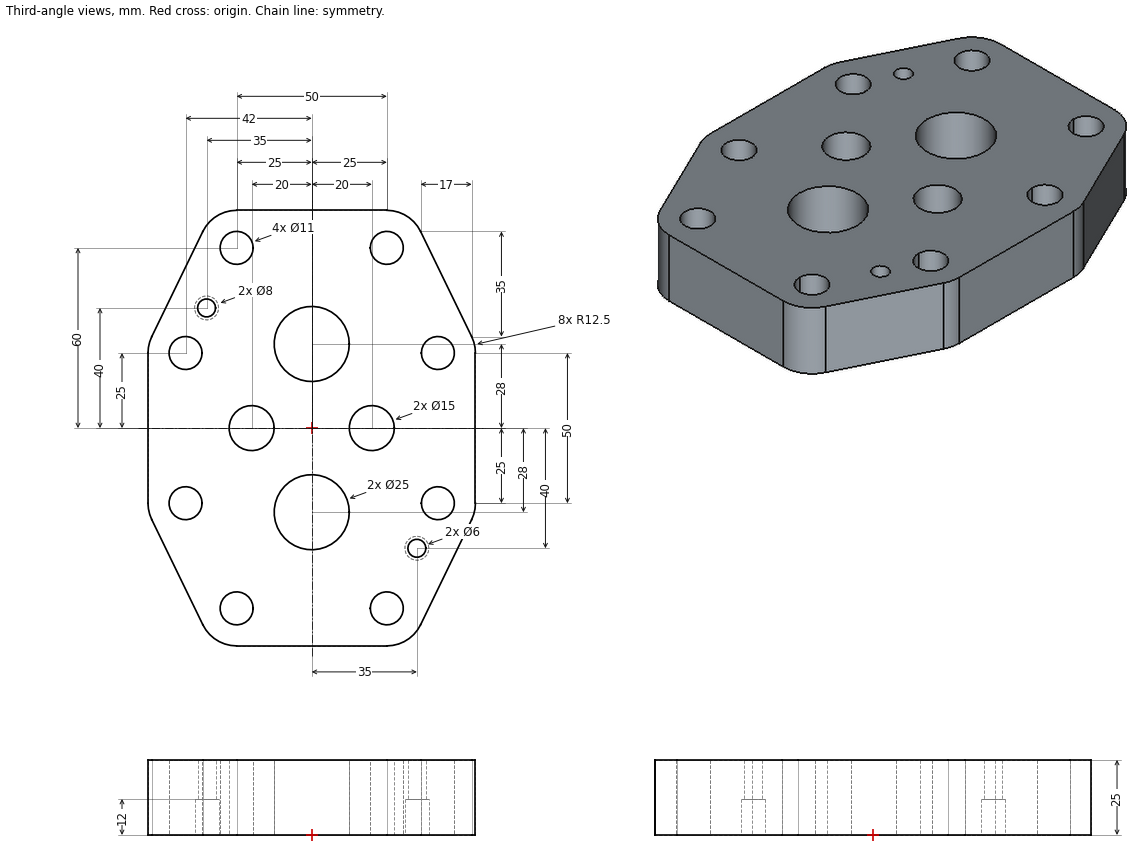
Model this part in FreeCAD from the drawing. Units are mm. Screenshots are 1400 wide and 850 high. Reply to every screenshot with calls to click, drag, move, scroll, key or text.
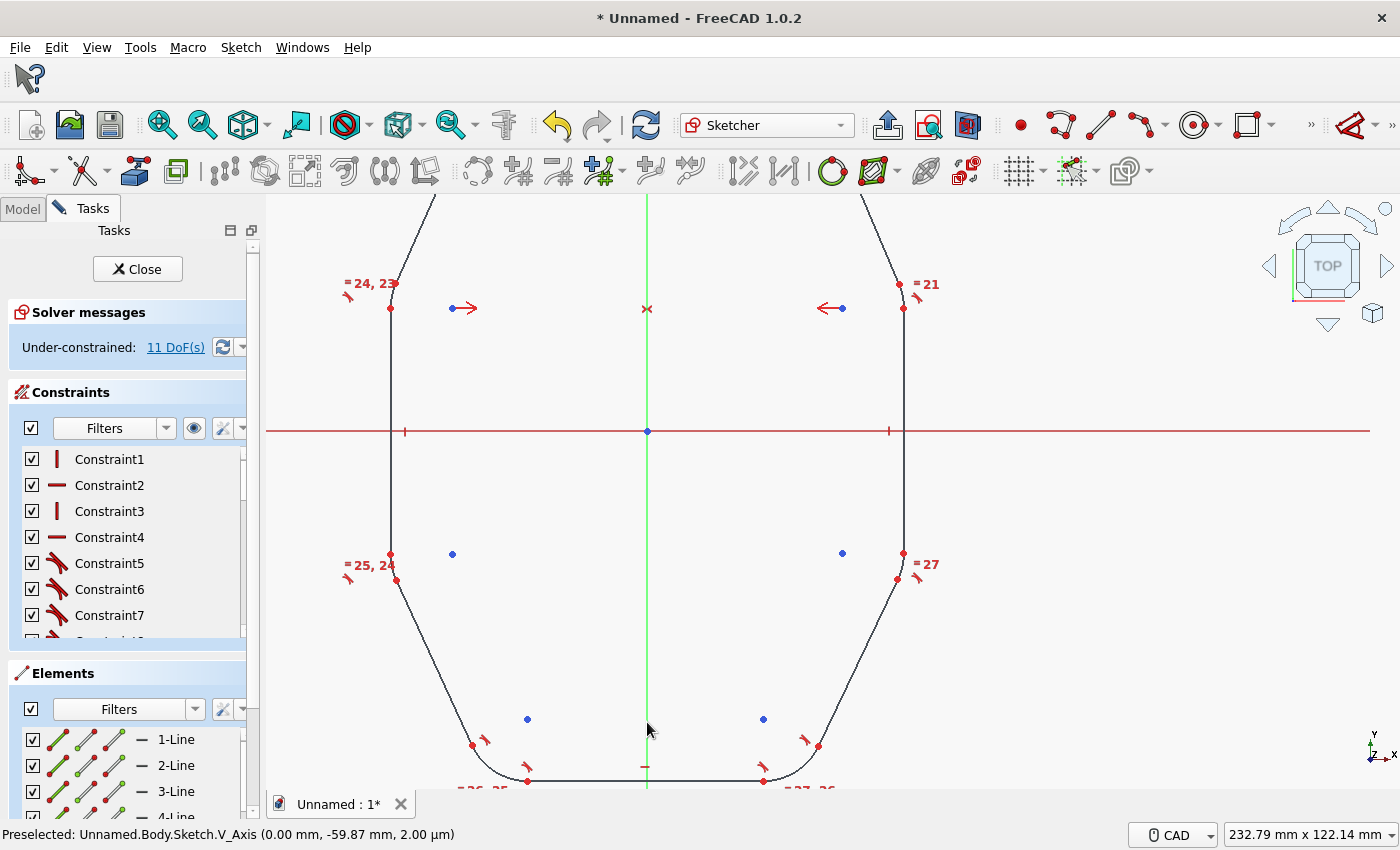
scroll(907, 565, down, 3)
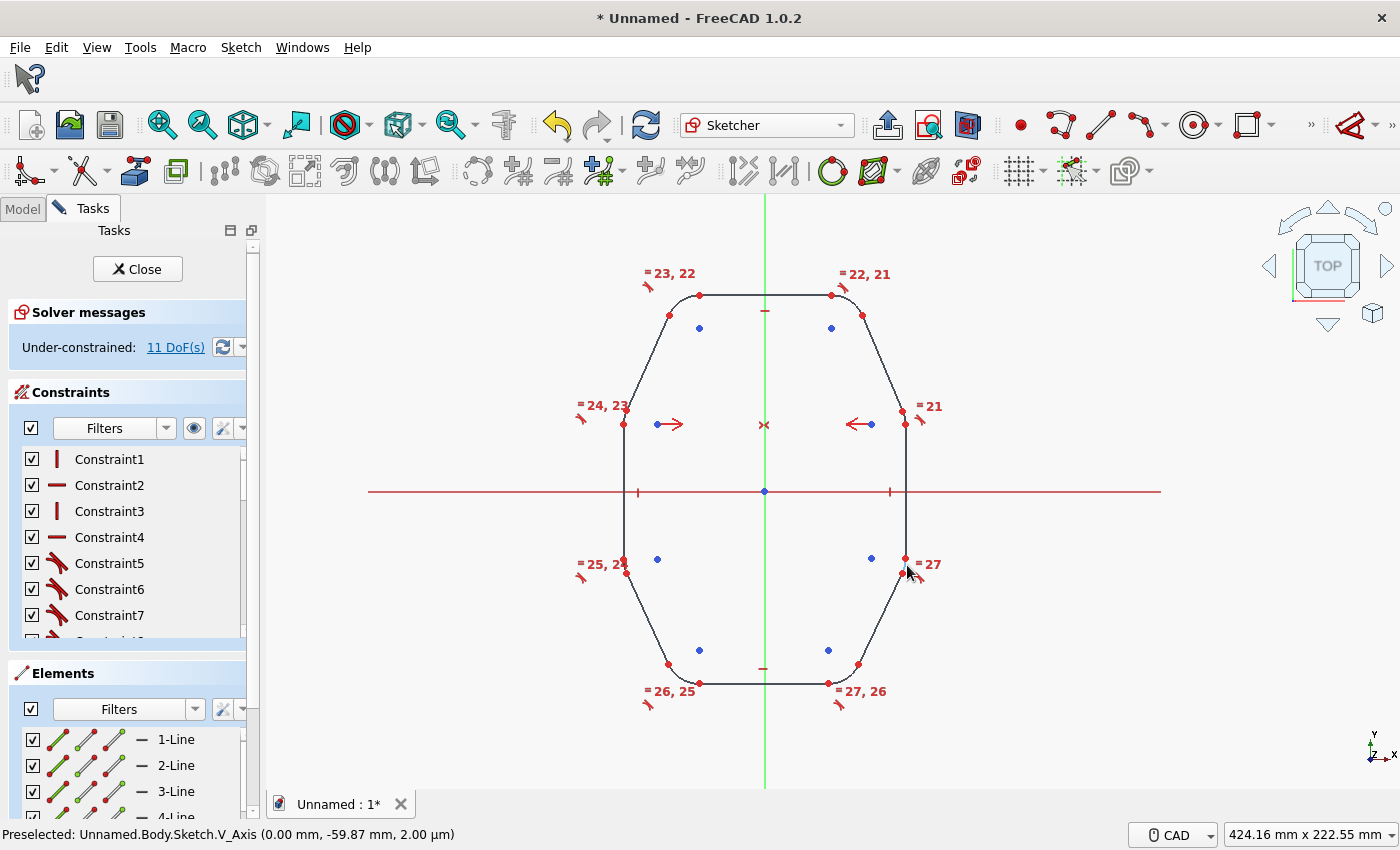
click(700, 329)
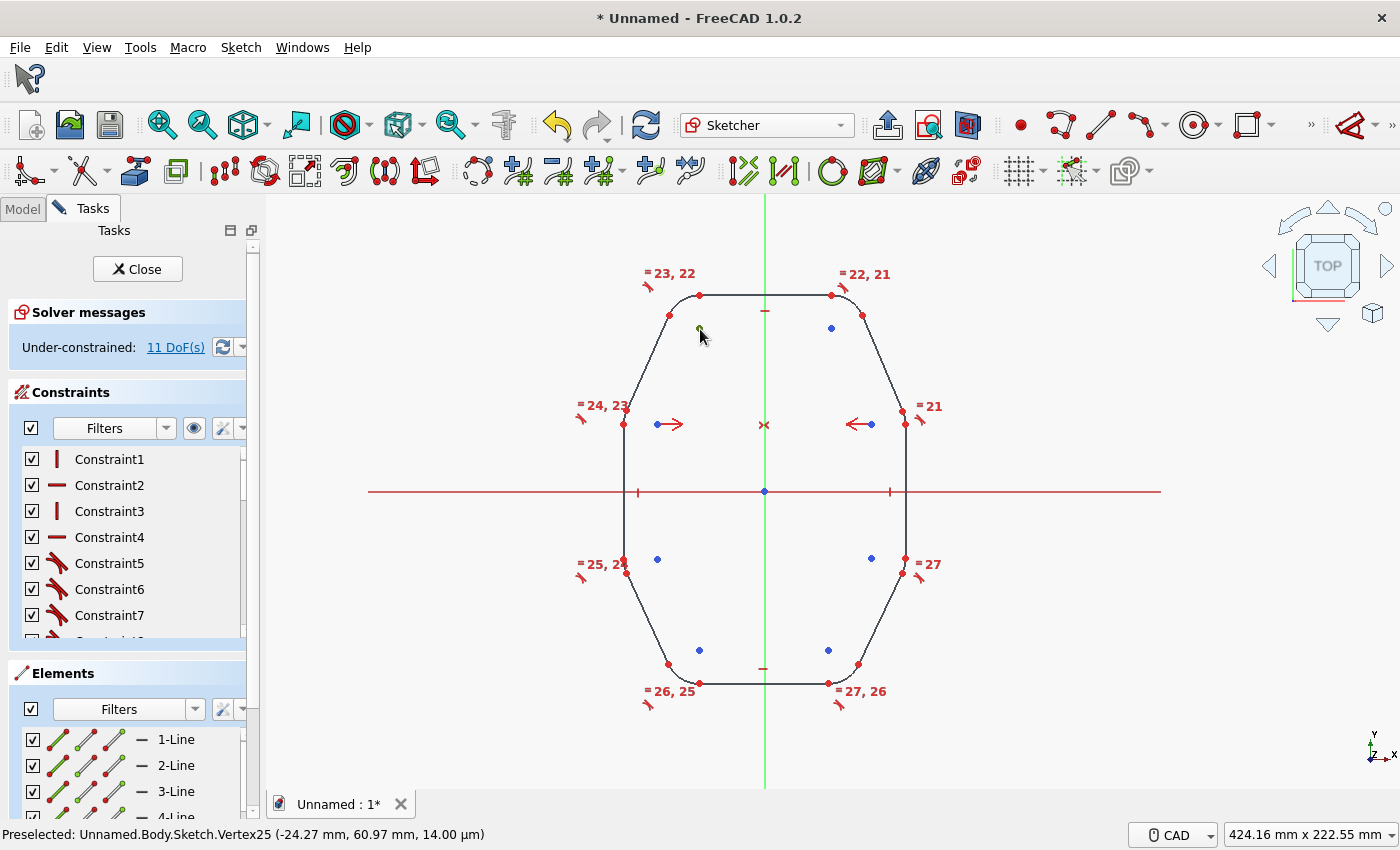
click(699, 650)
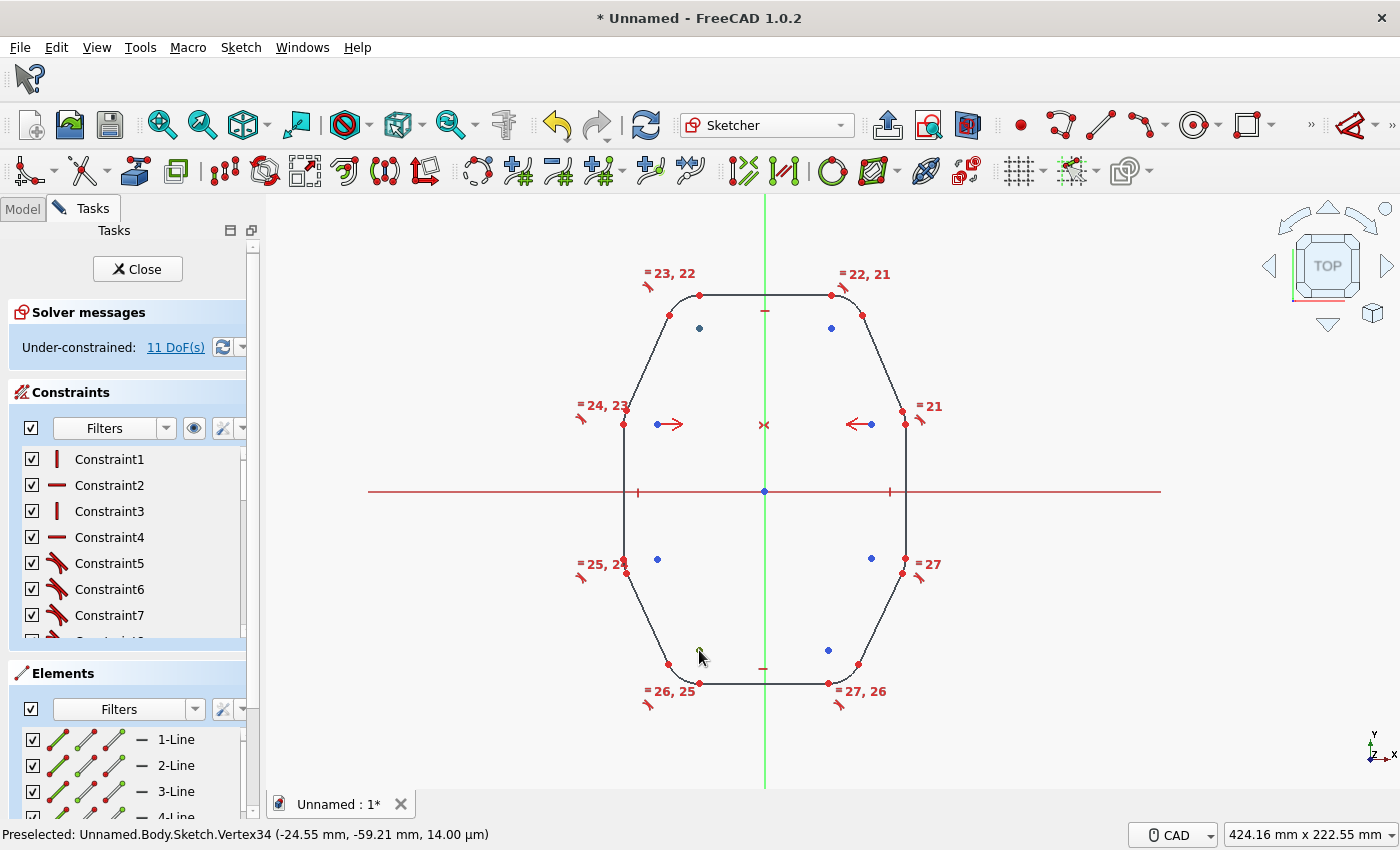
click(428, 492)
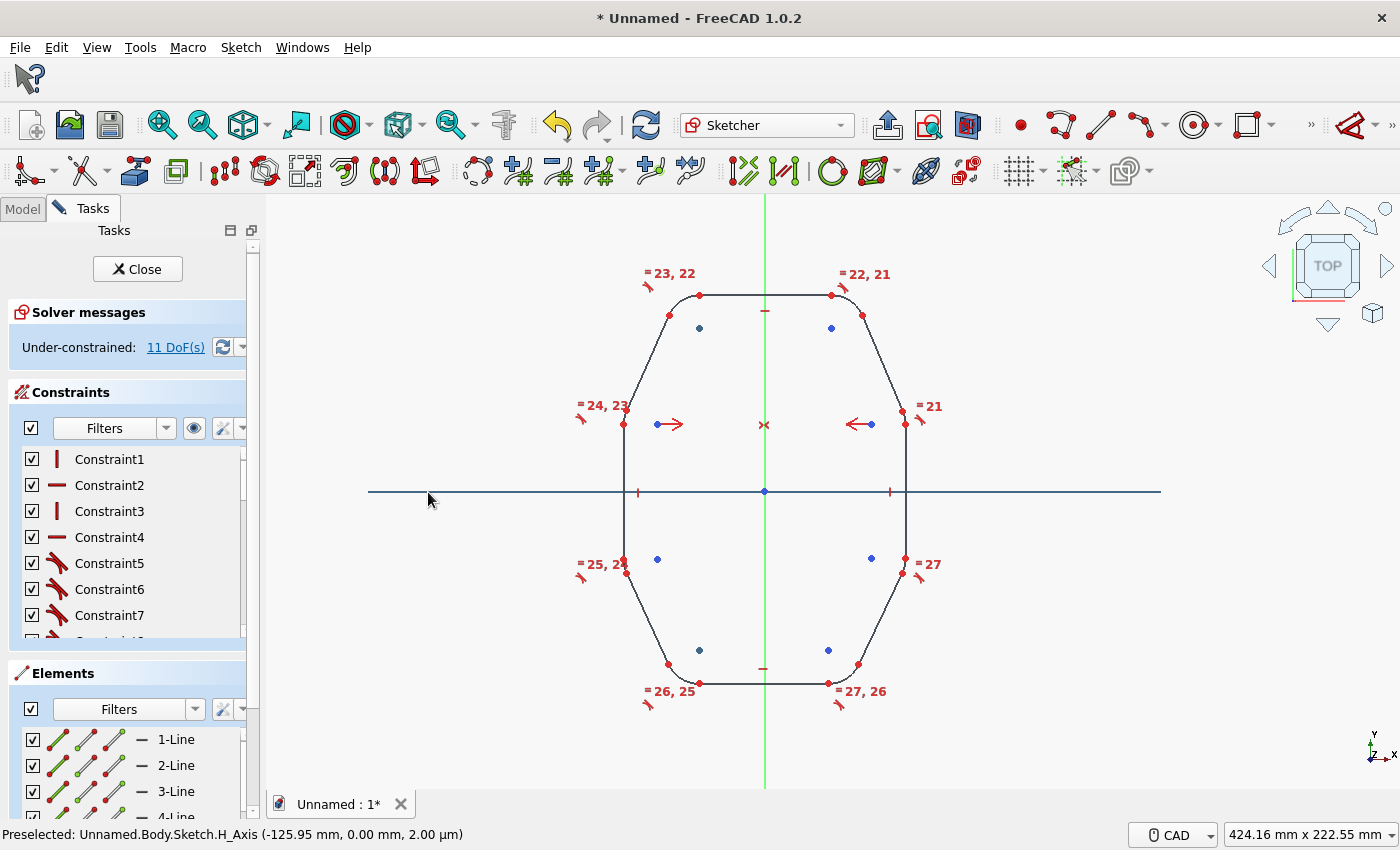
key(s)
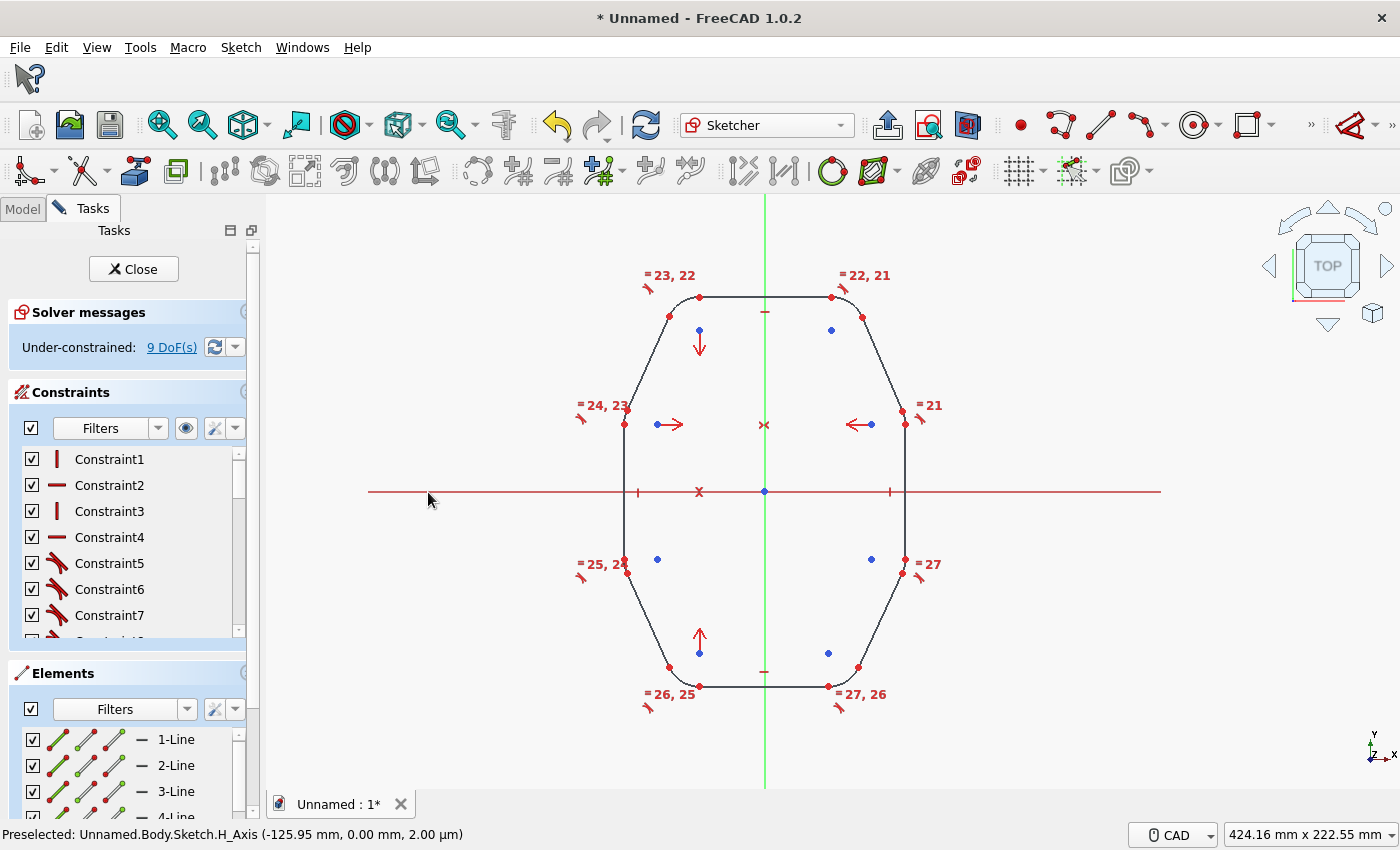
key(d)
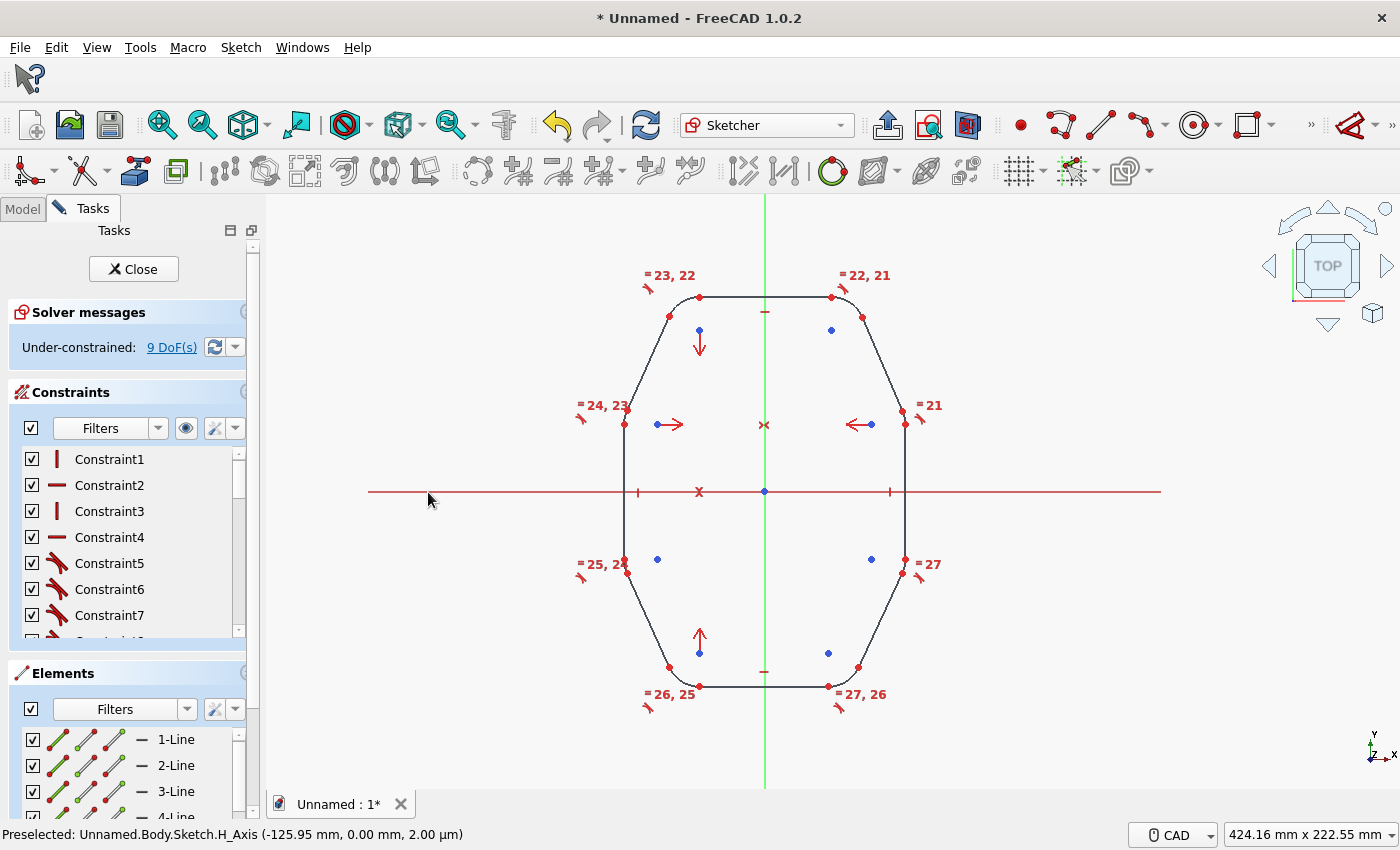
scroll(905, 418, up, 4)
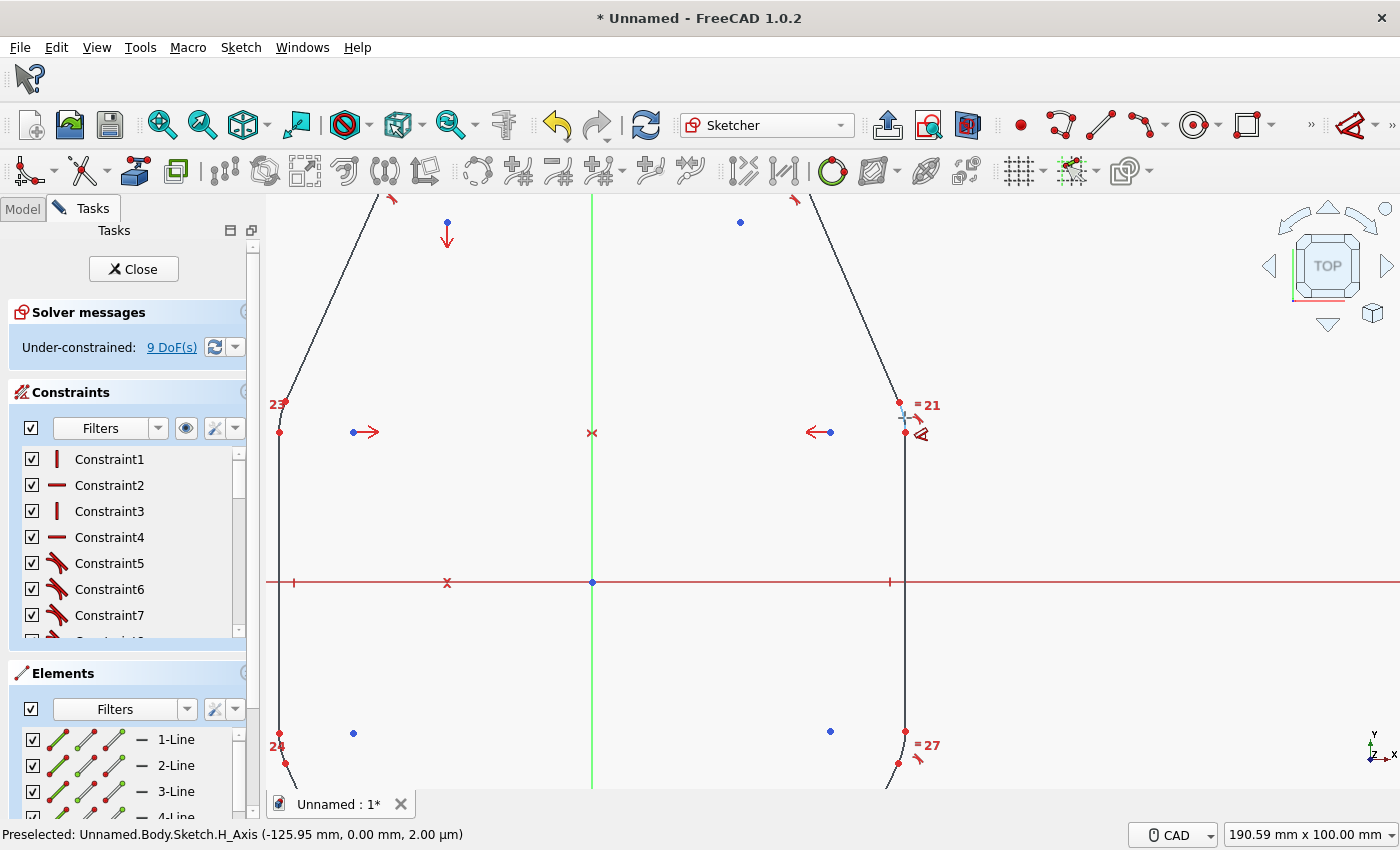
click(904, 417)
click(935, 411)